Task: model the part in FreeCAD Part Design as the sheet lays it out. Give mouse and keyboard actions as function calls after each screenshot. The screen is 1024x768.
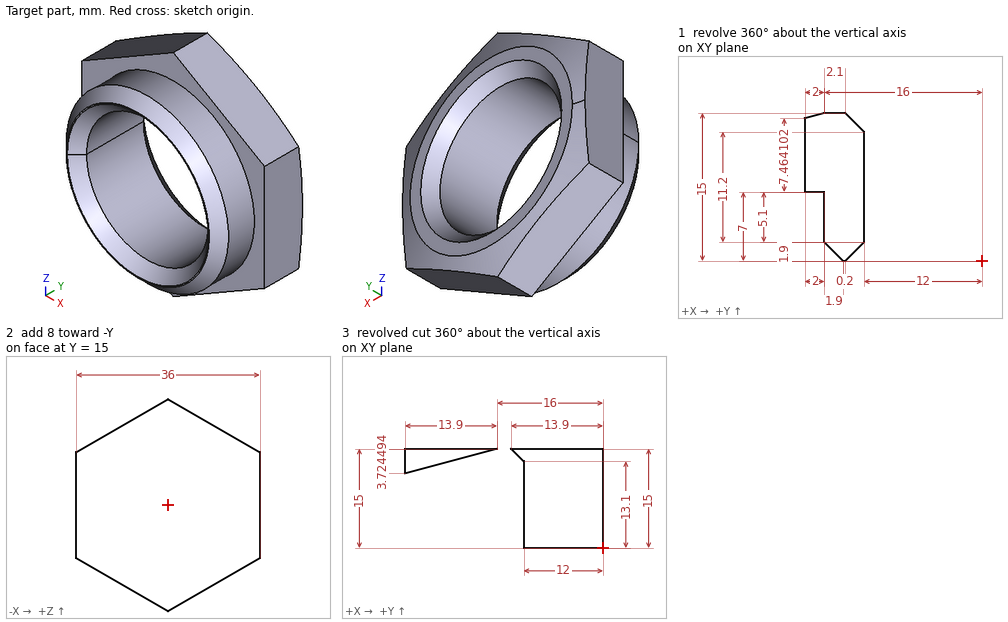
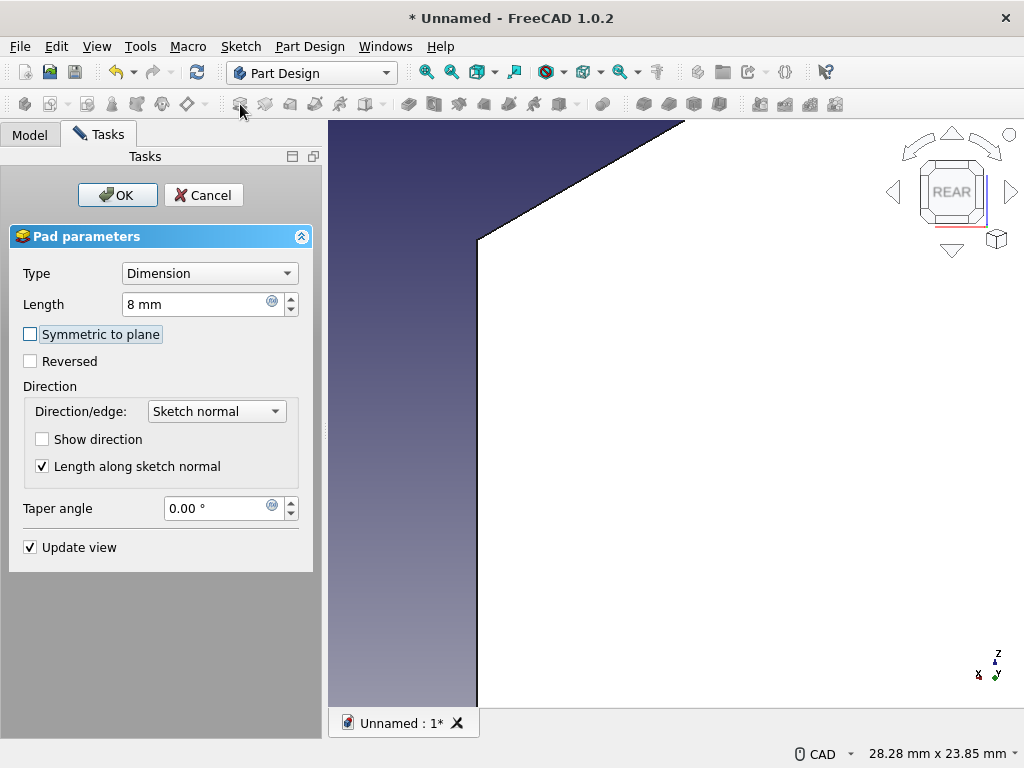
click(31, 361)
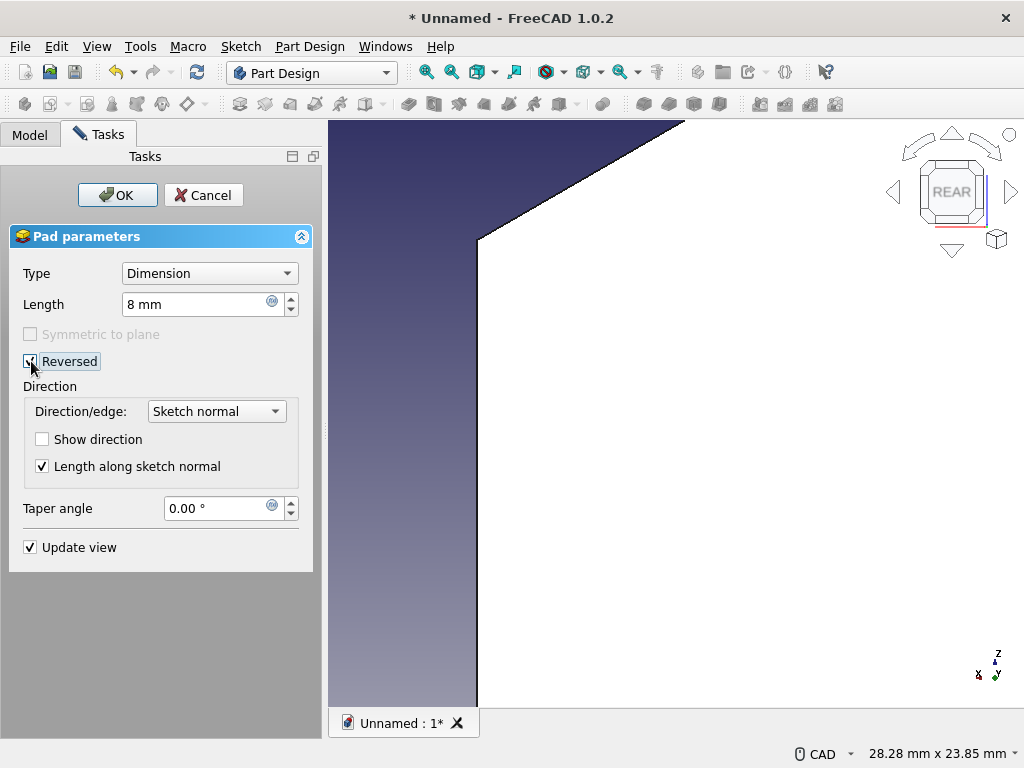
click(118, 195)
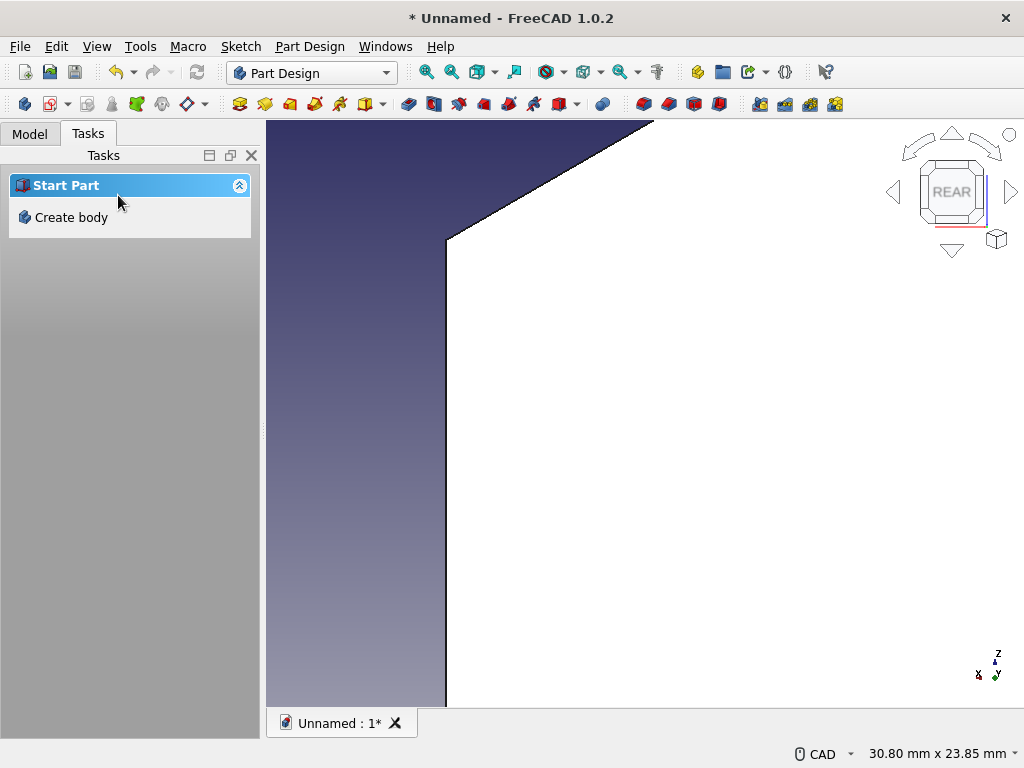
click(427, 72)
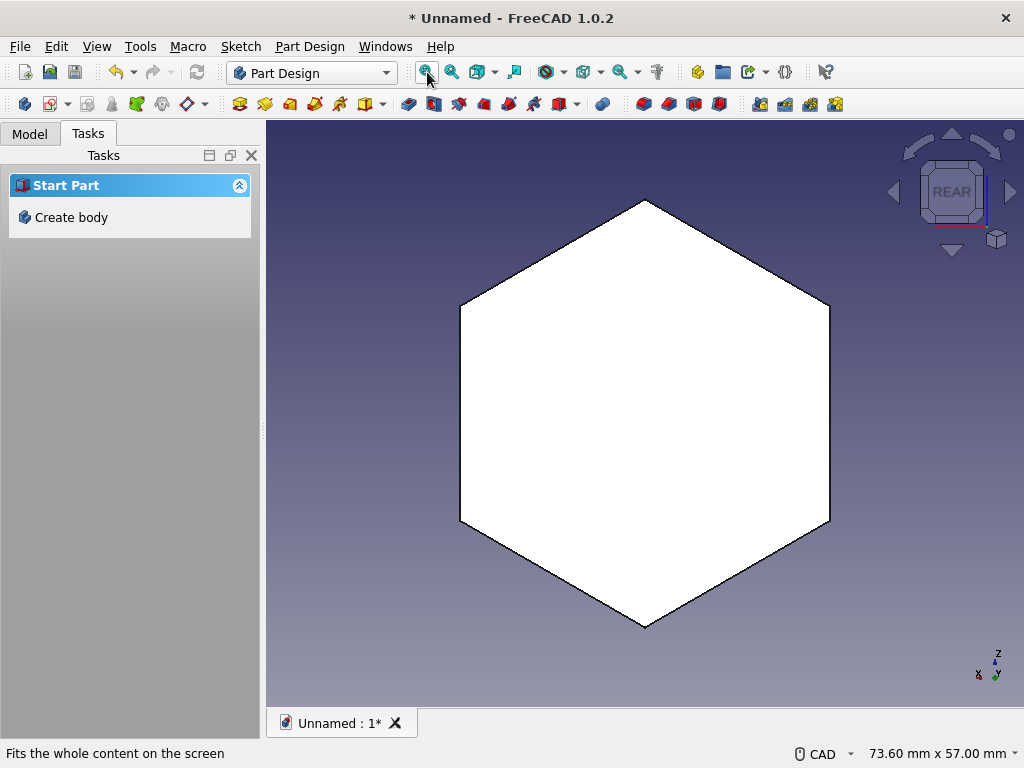
click(50, 104)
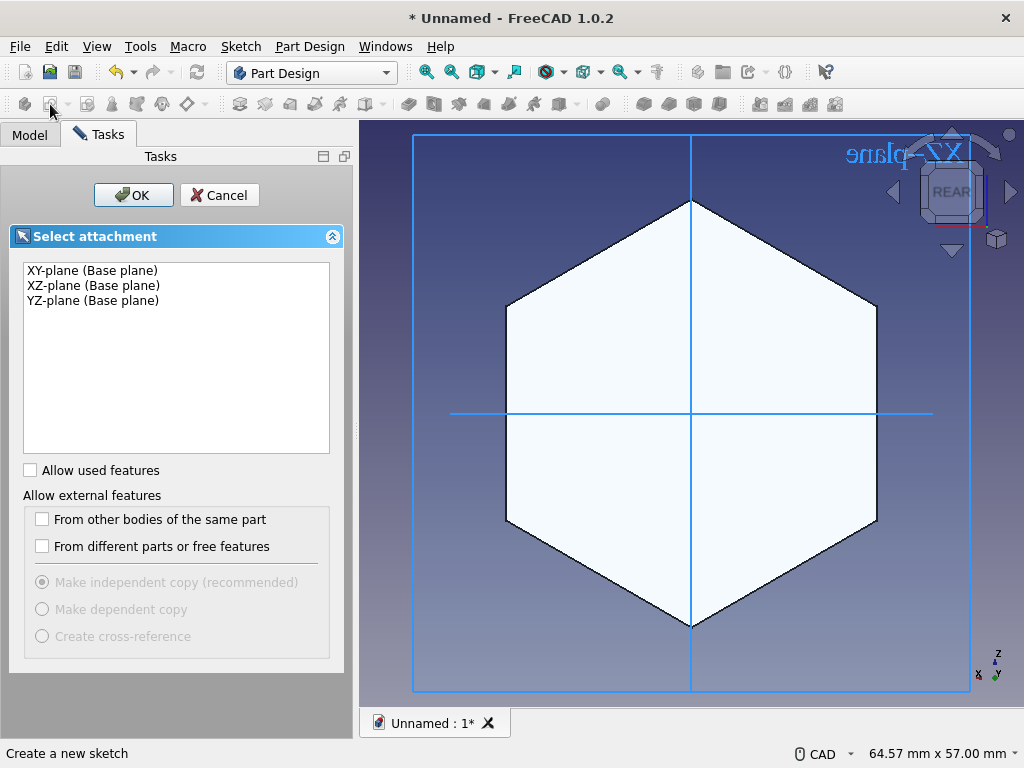
click(84, 270)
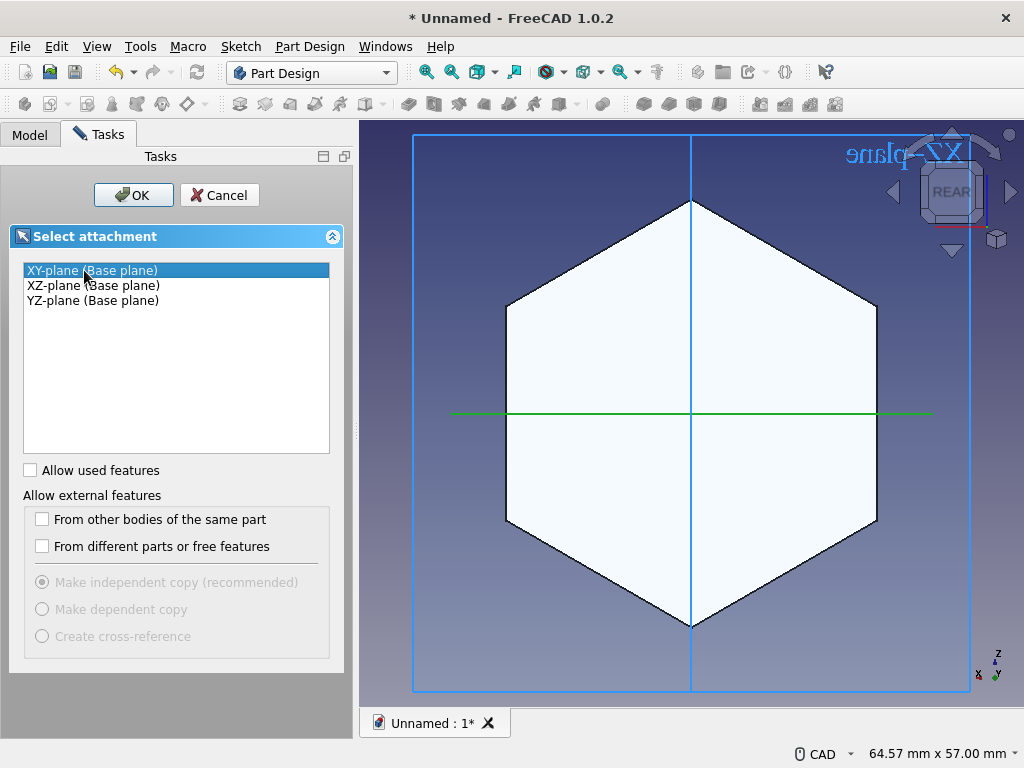
click(134, 195)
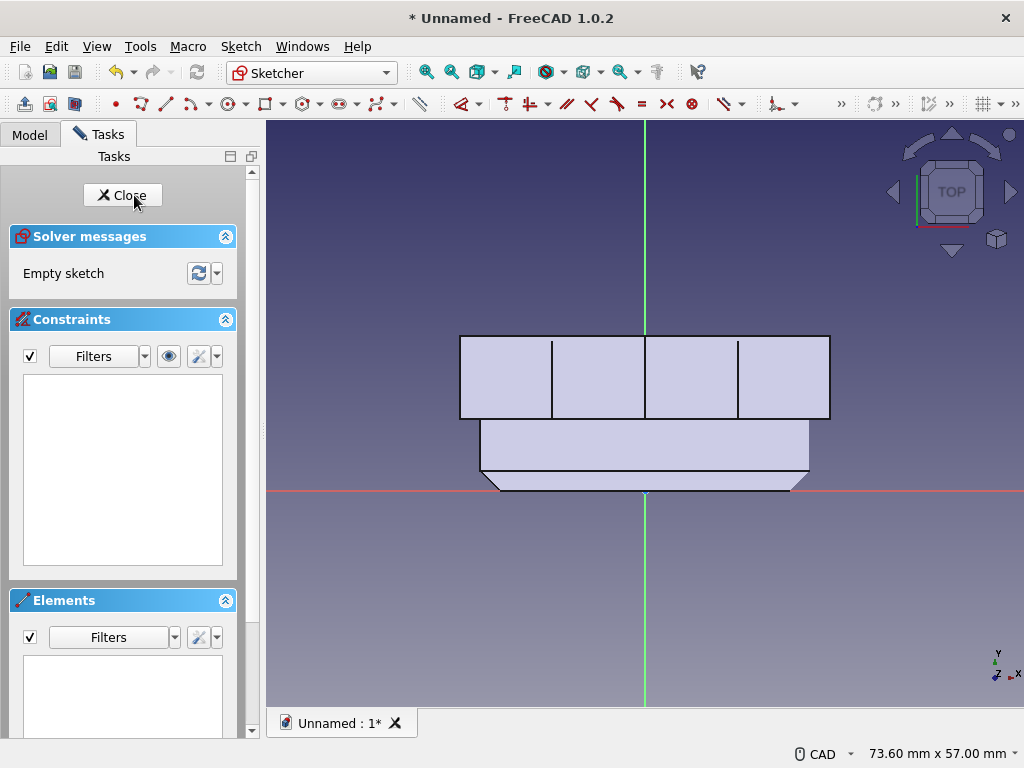
click(75, 104)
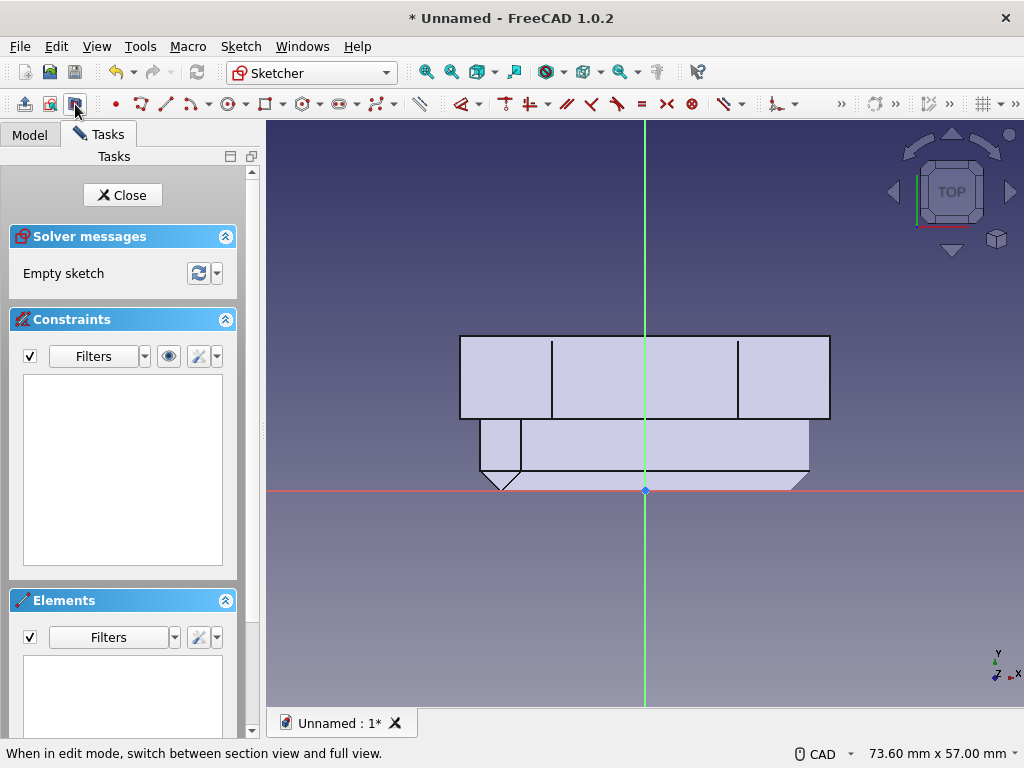
click(141, 104)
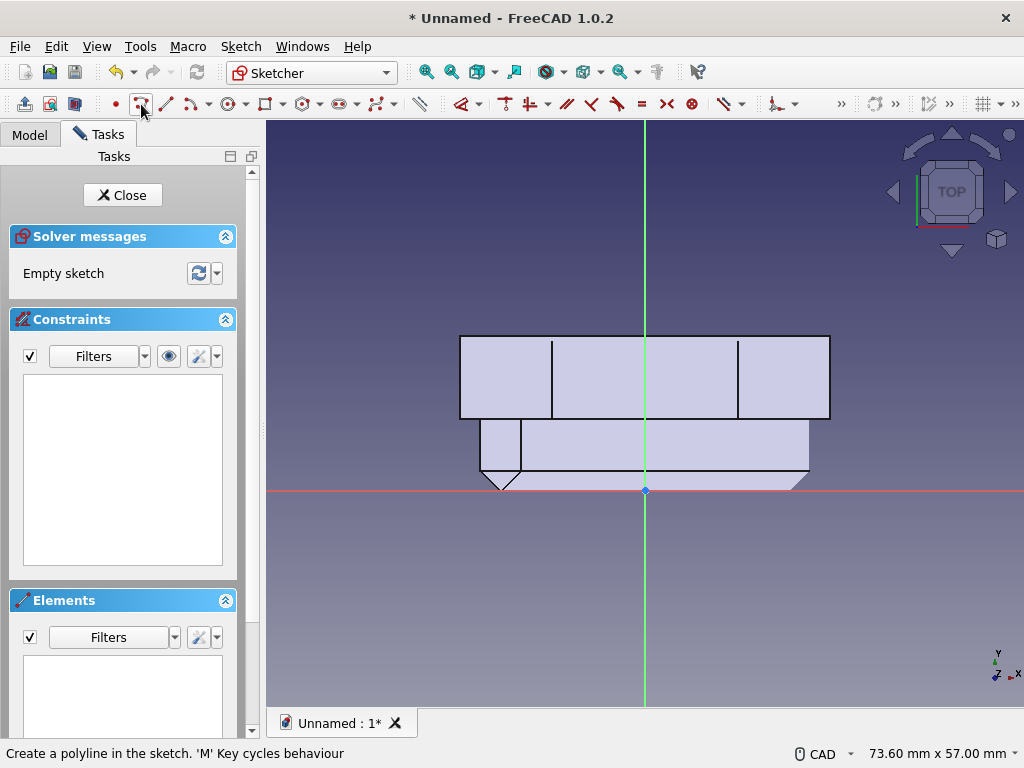
click(480, 336)
click(337, 336)
click(337, 375)
click(480, 337)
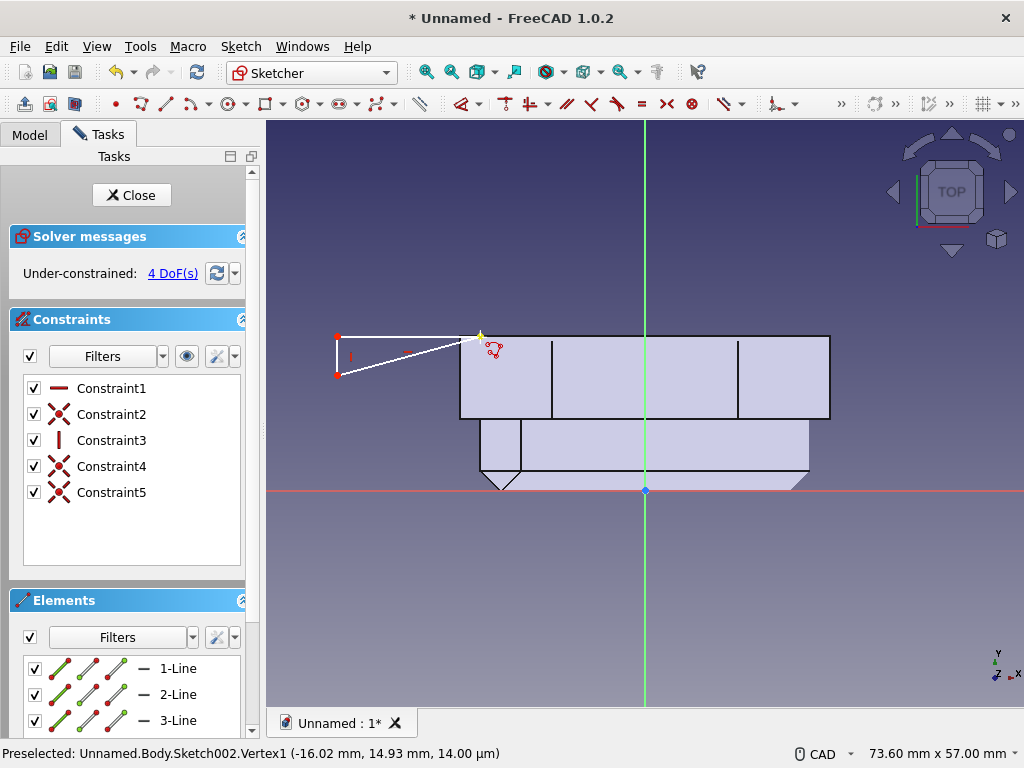
click(645, 491)
click(636, 336)
click(502, 336)
click(521, 356)
click(521, 482)
click(645, 491)
key(Escape)
key(Escape)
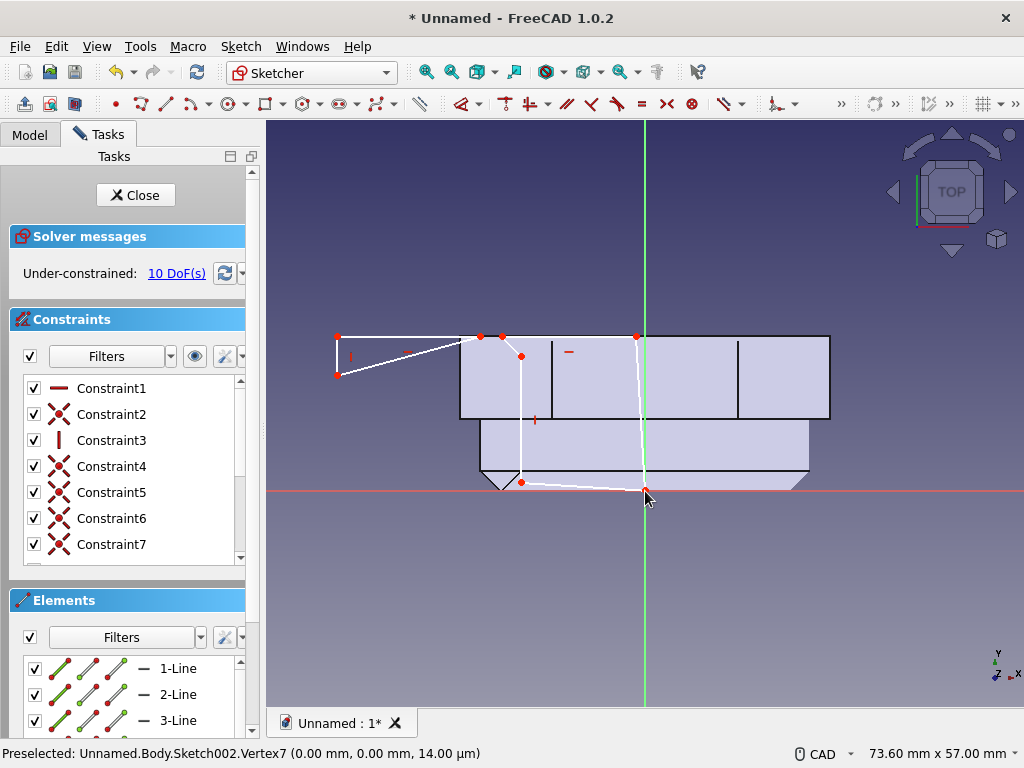
click(642, 445)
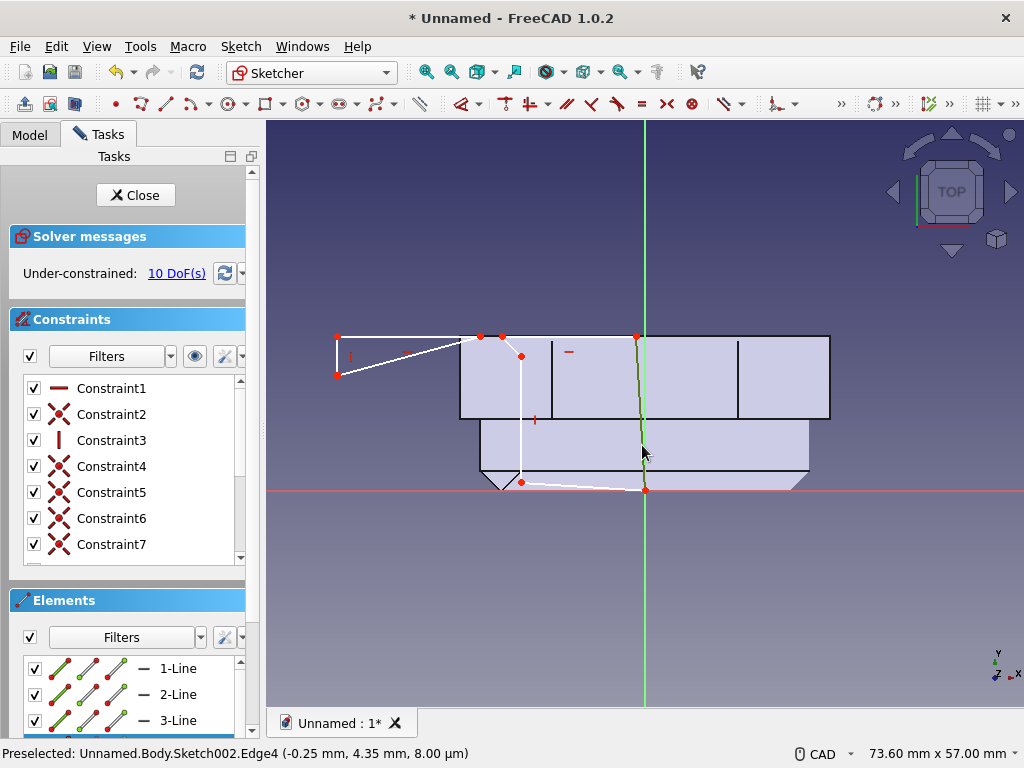
click(548, 104)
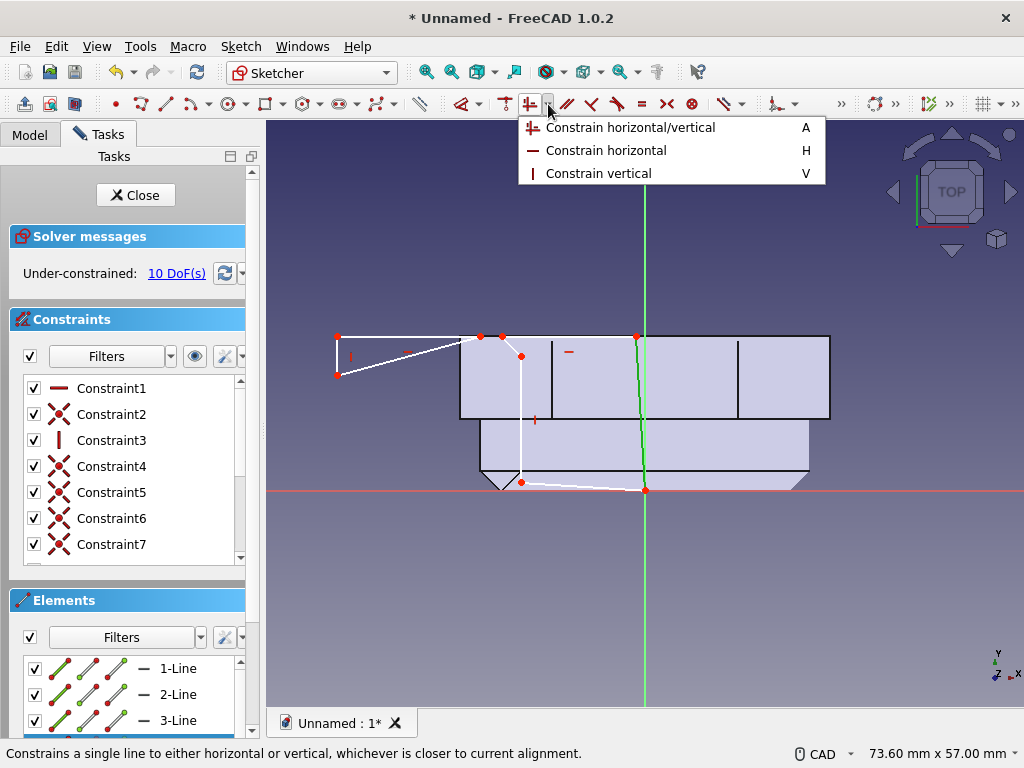
click(672, 174)